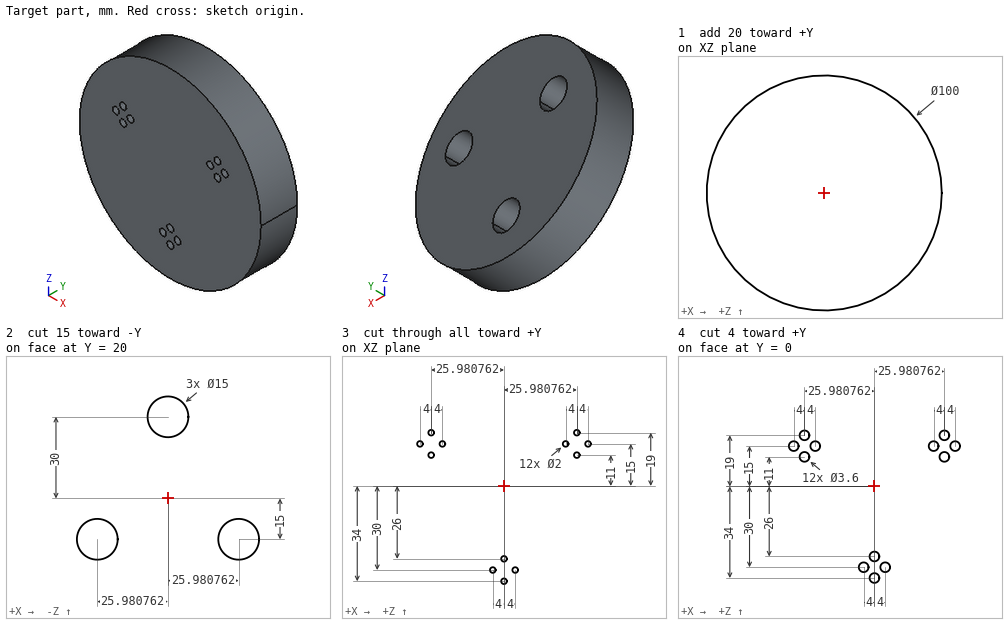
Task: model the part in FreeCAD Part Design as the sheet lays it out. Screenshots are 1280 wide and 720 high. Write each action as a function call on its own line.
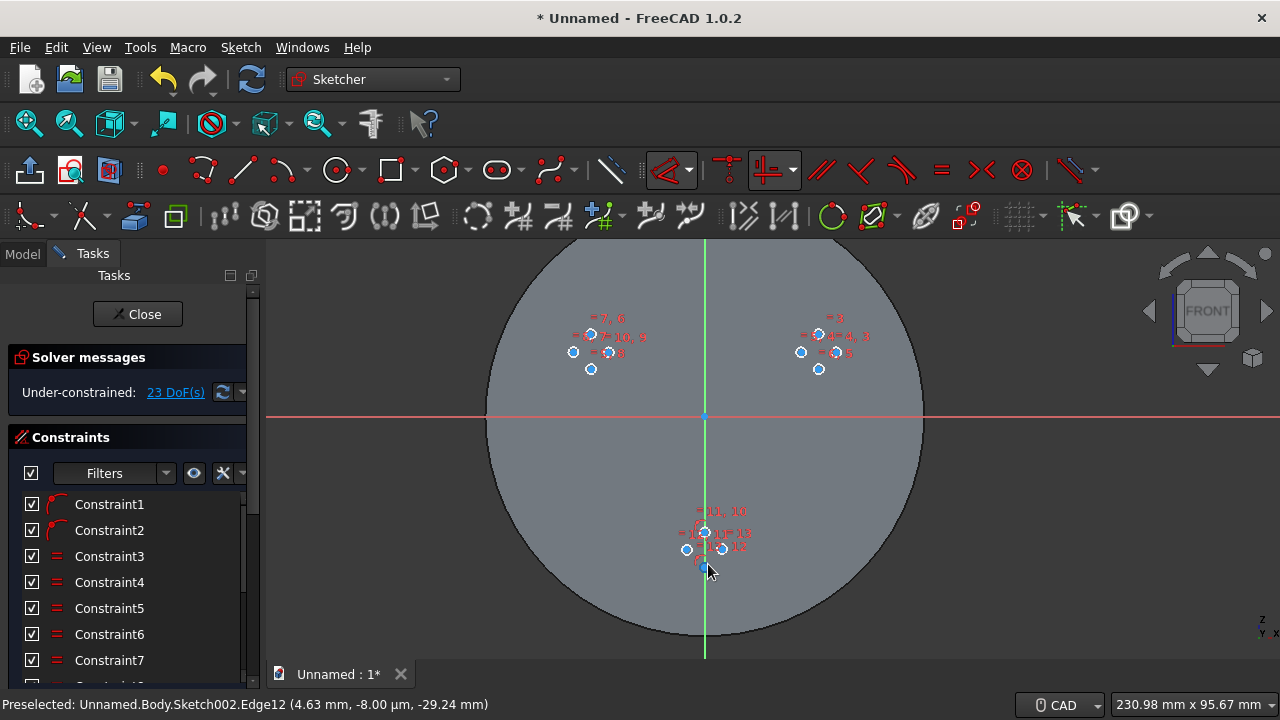
click(836, 352)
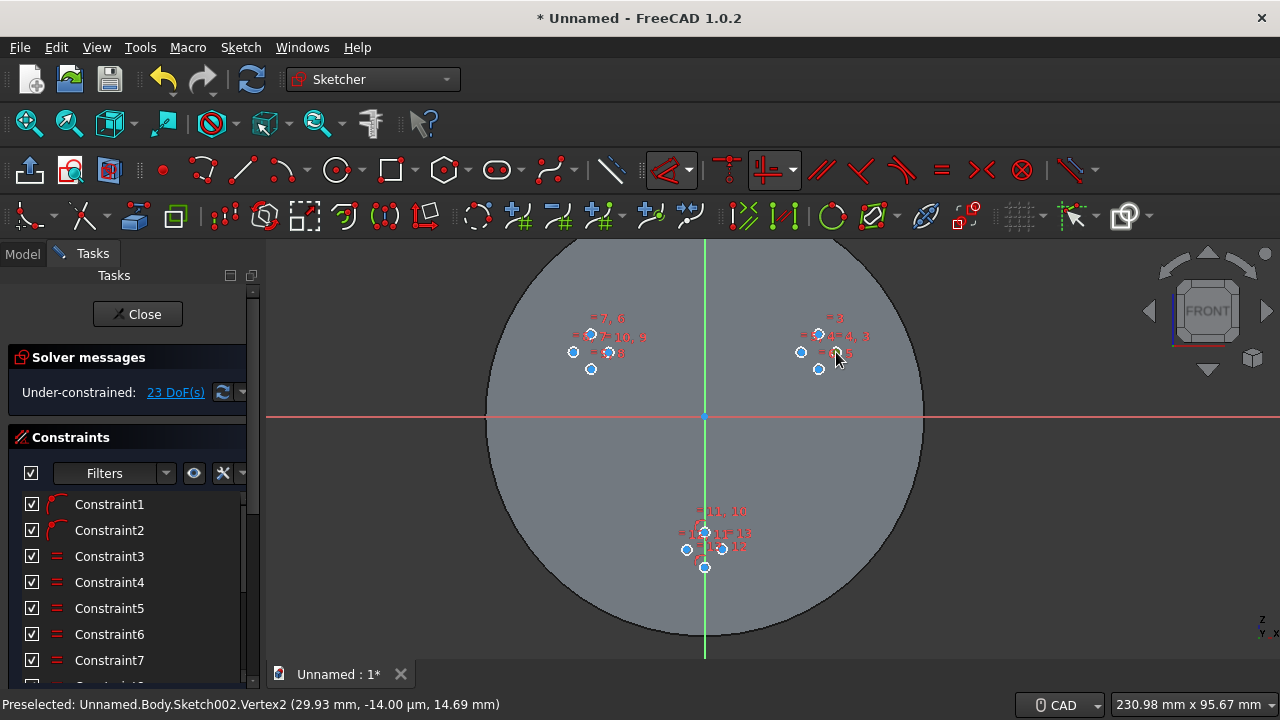
click(801, 352)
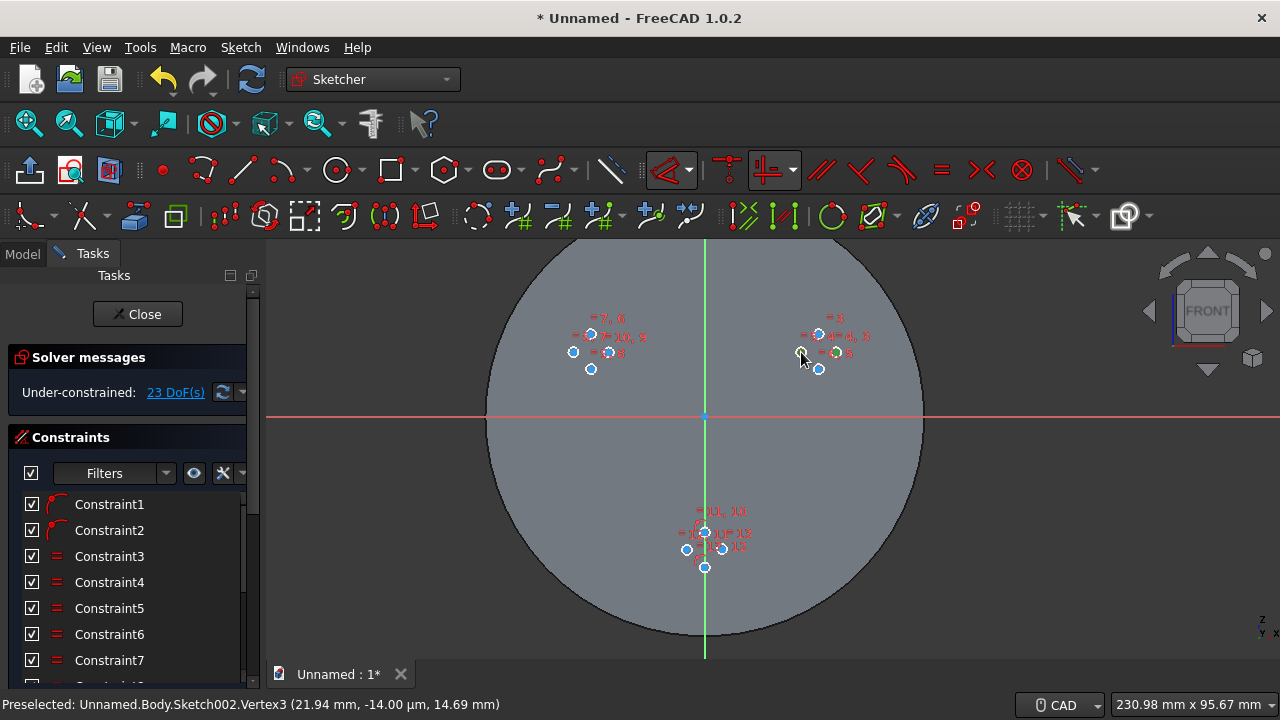
click(796, 170)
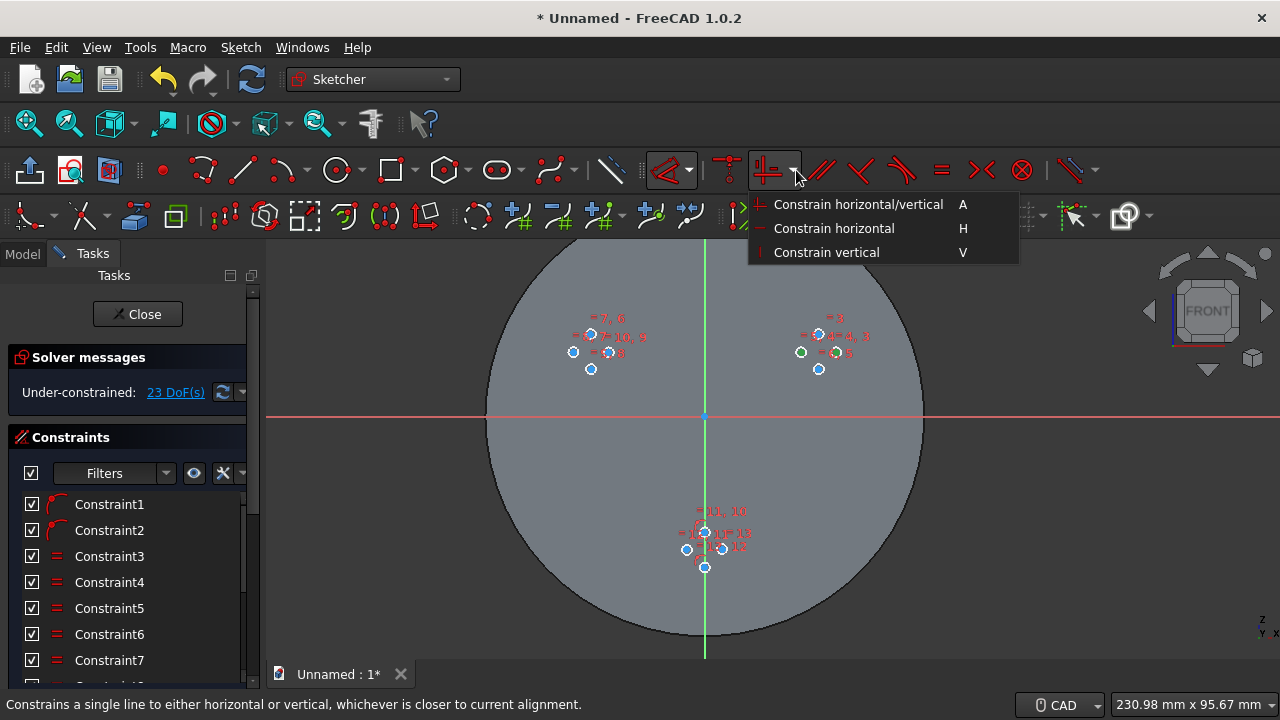
click(884, 228)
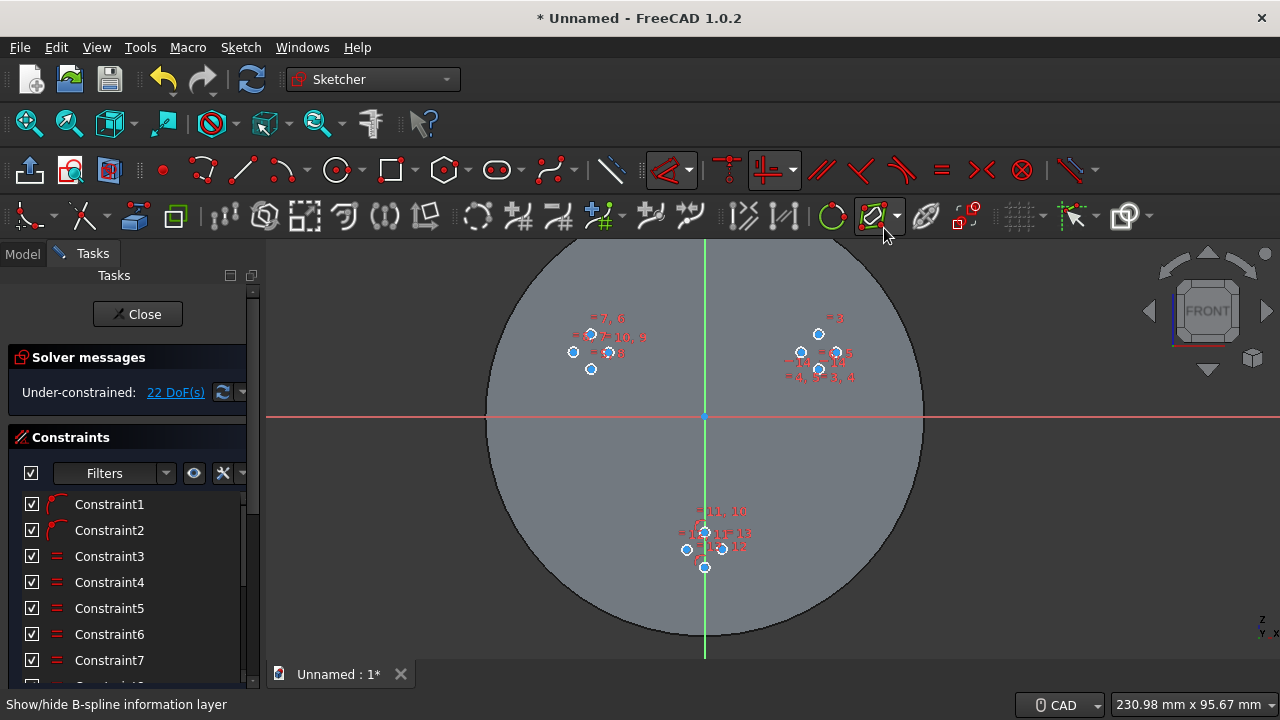
click(819, 334)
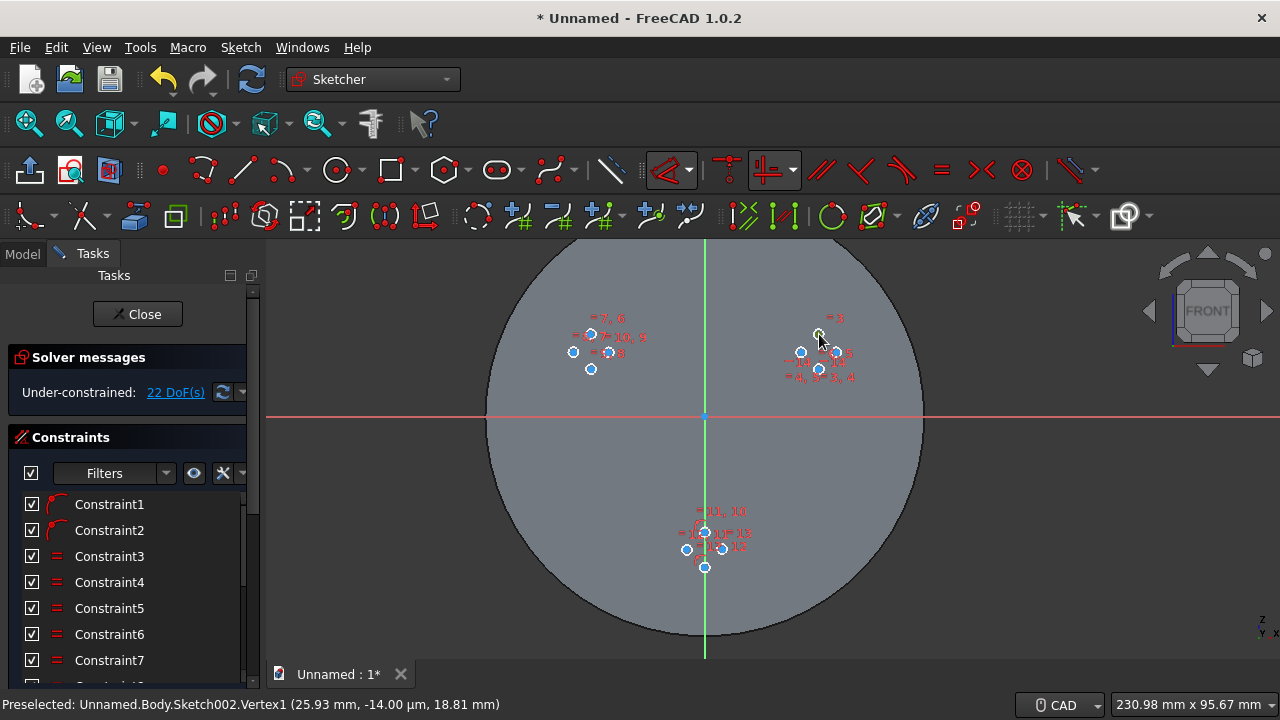
click(821, 371)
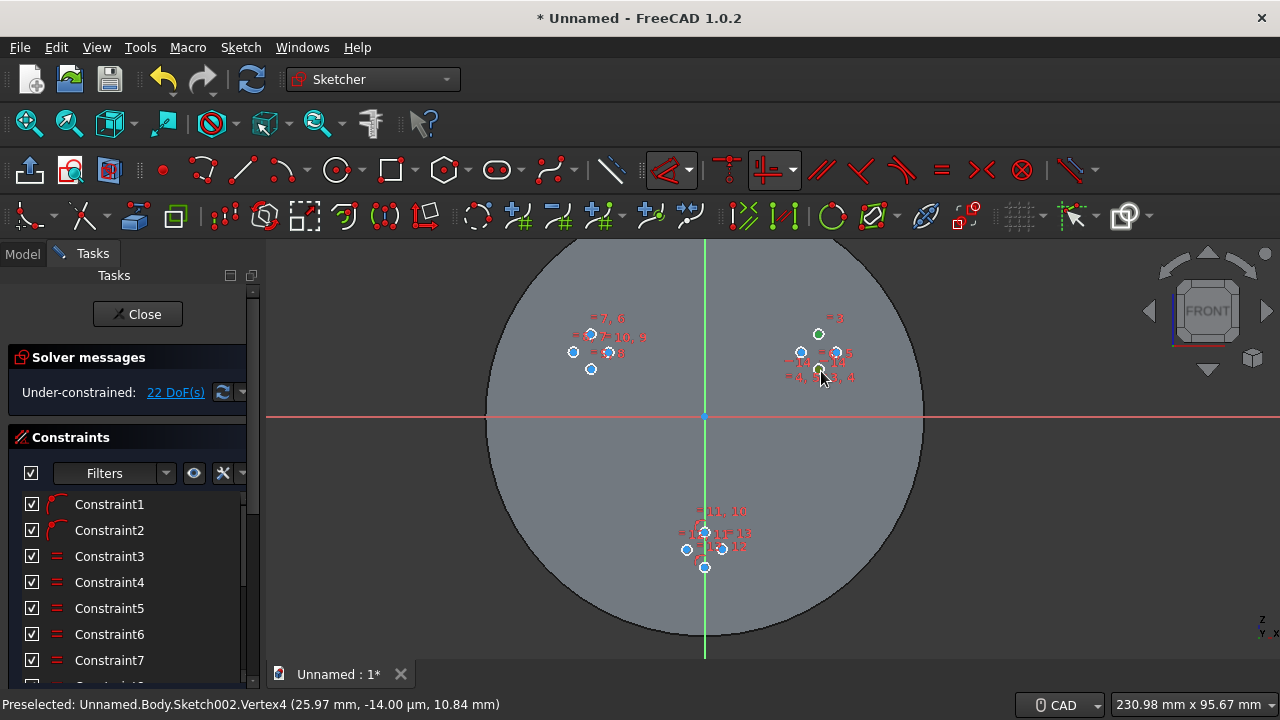
key(v)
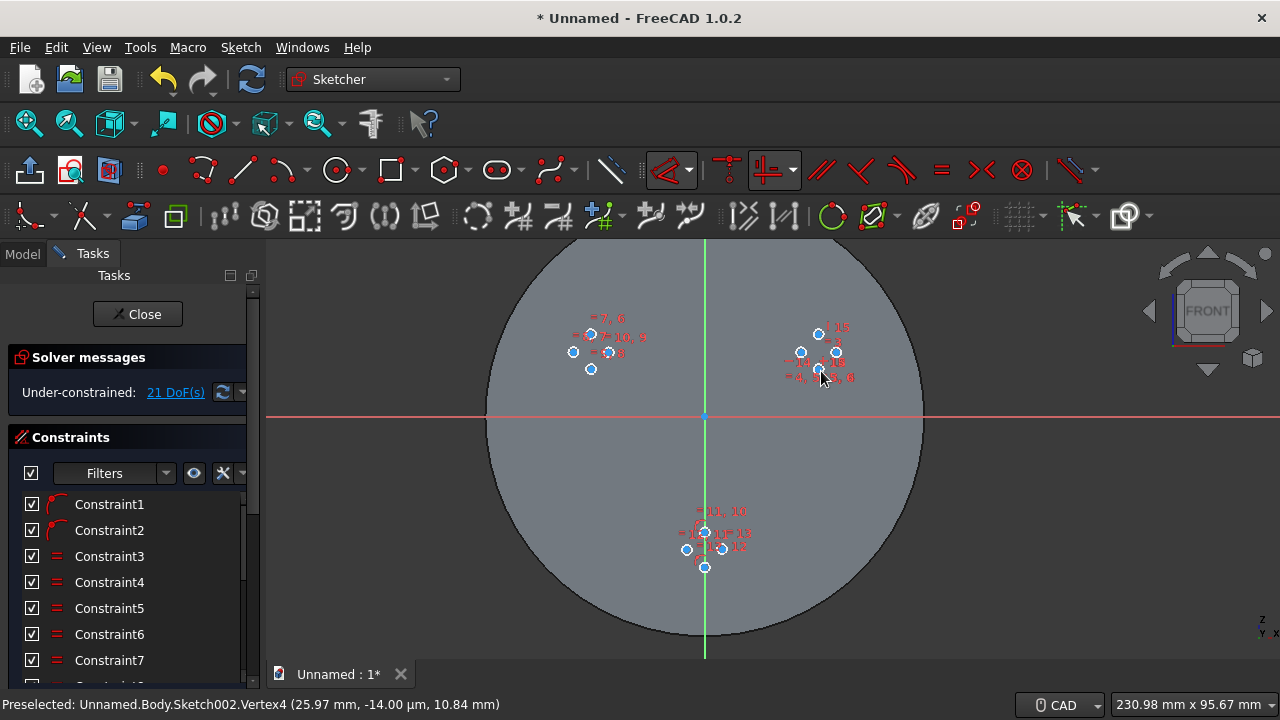
click(819, 334)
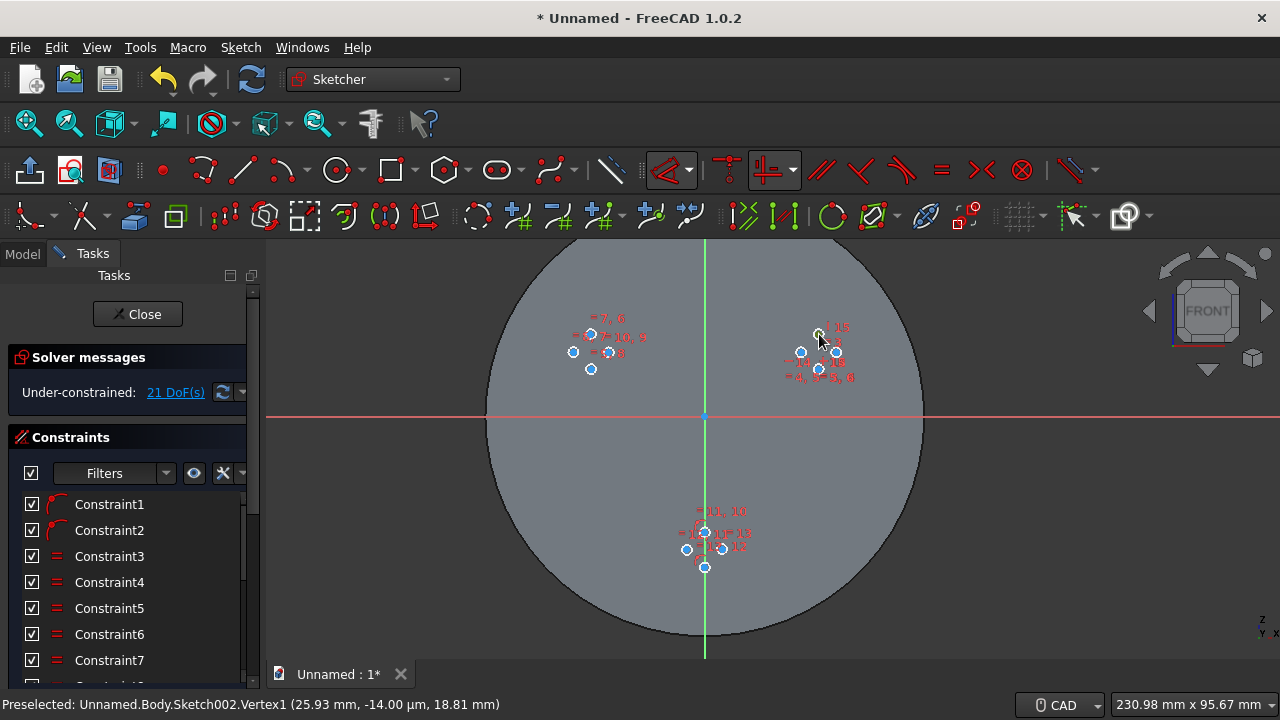
click(591, 334)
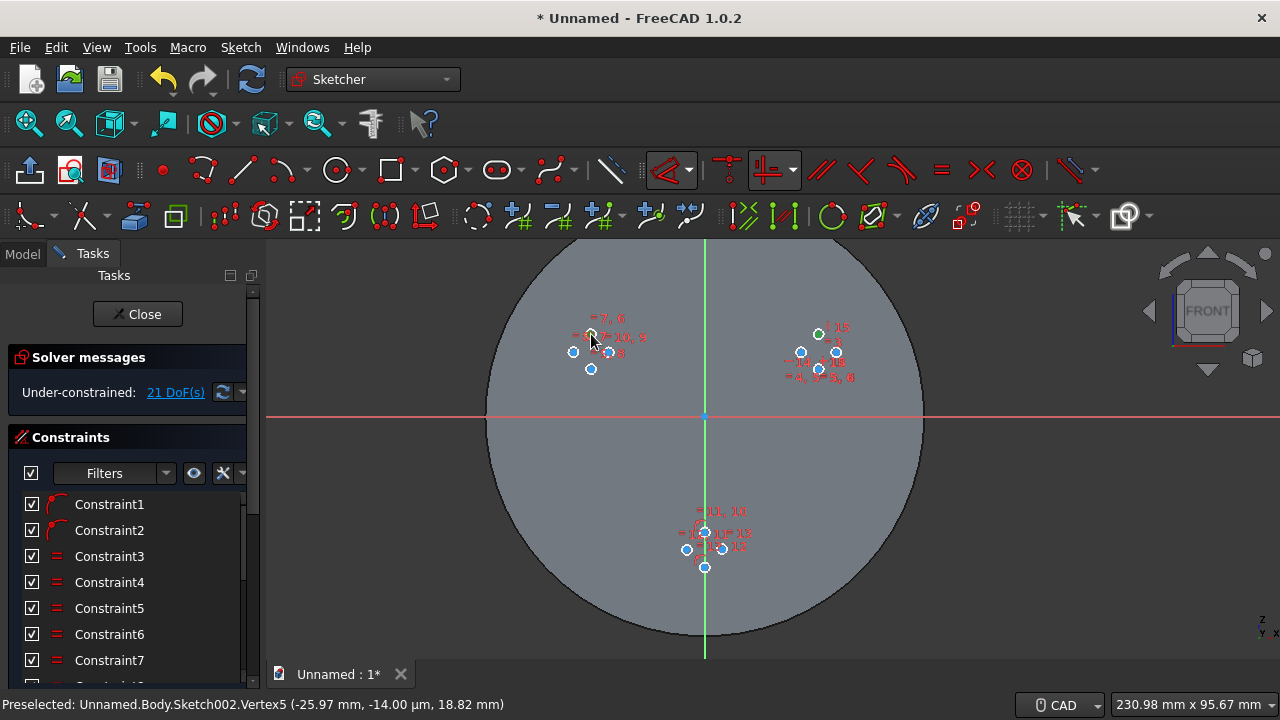
key(h)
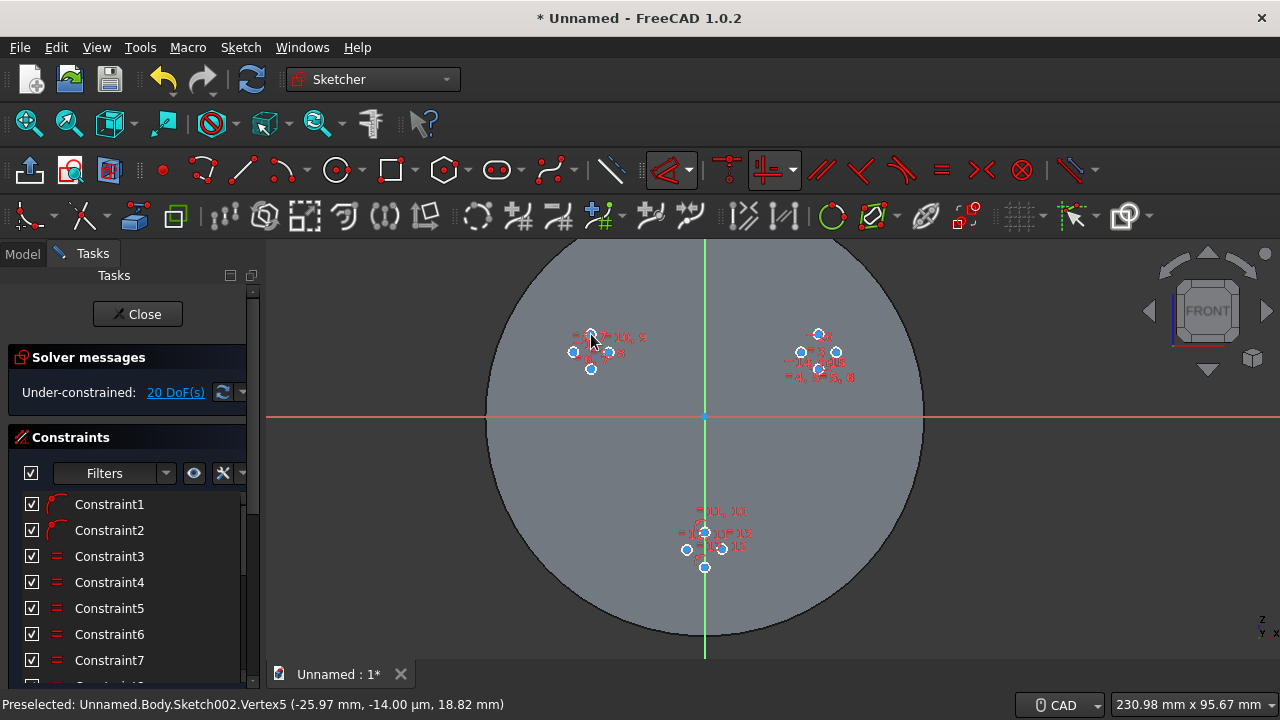
click(801, 352)